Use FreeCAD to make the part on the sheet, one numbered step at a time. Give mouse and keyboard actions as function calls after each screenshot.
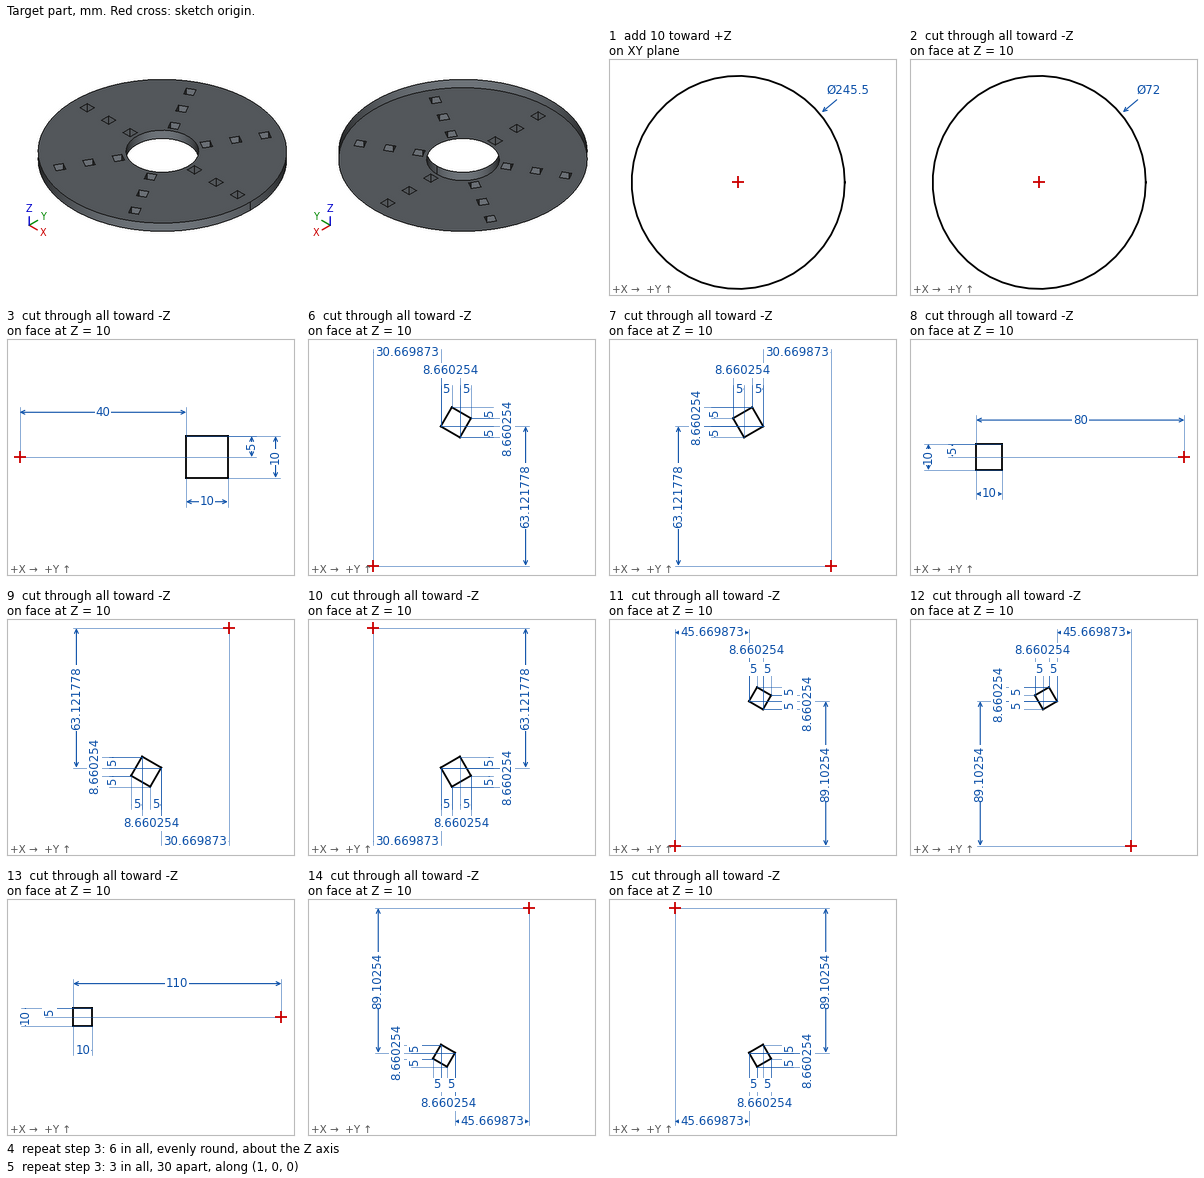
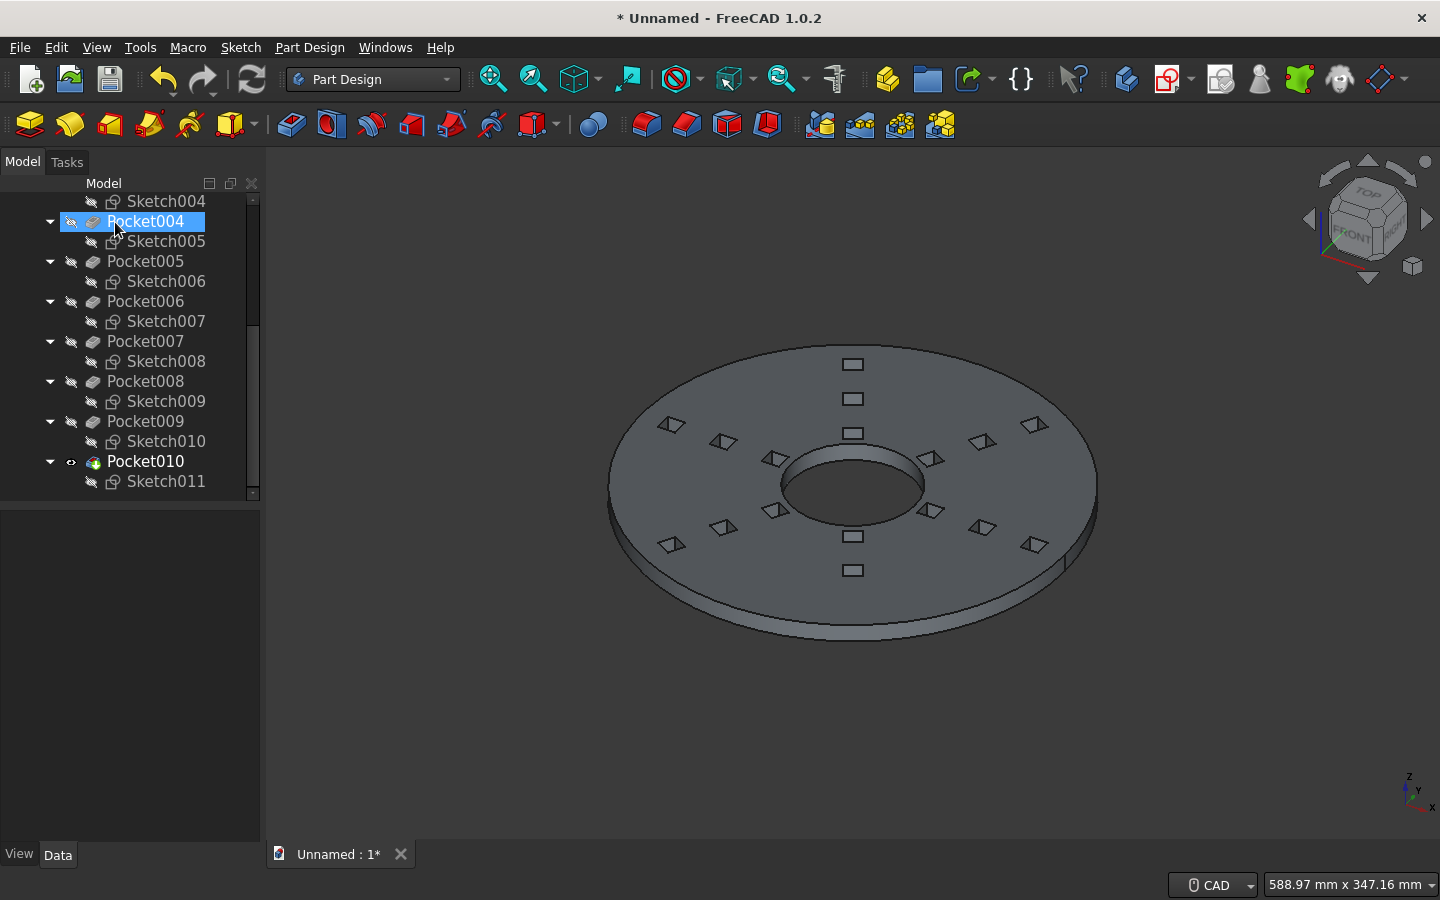
click(923, 414)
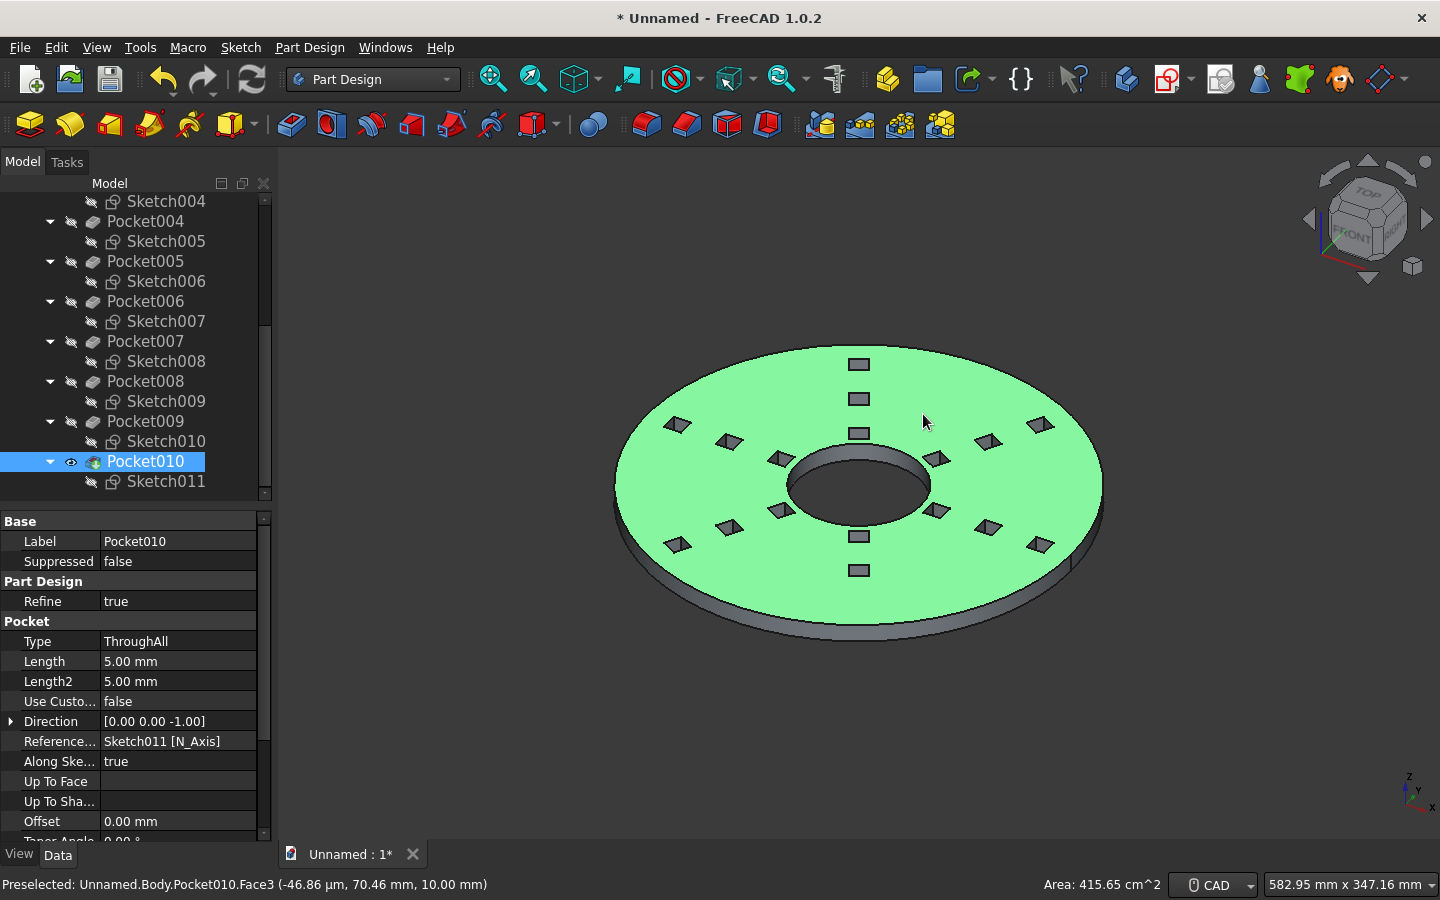
click(1168, 80)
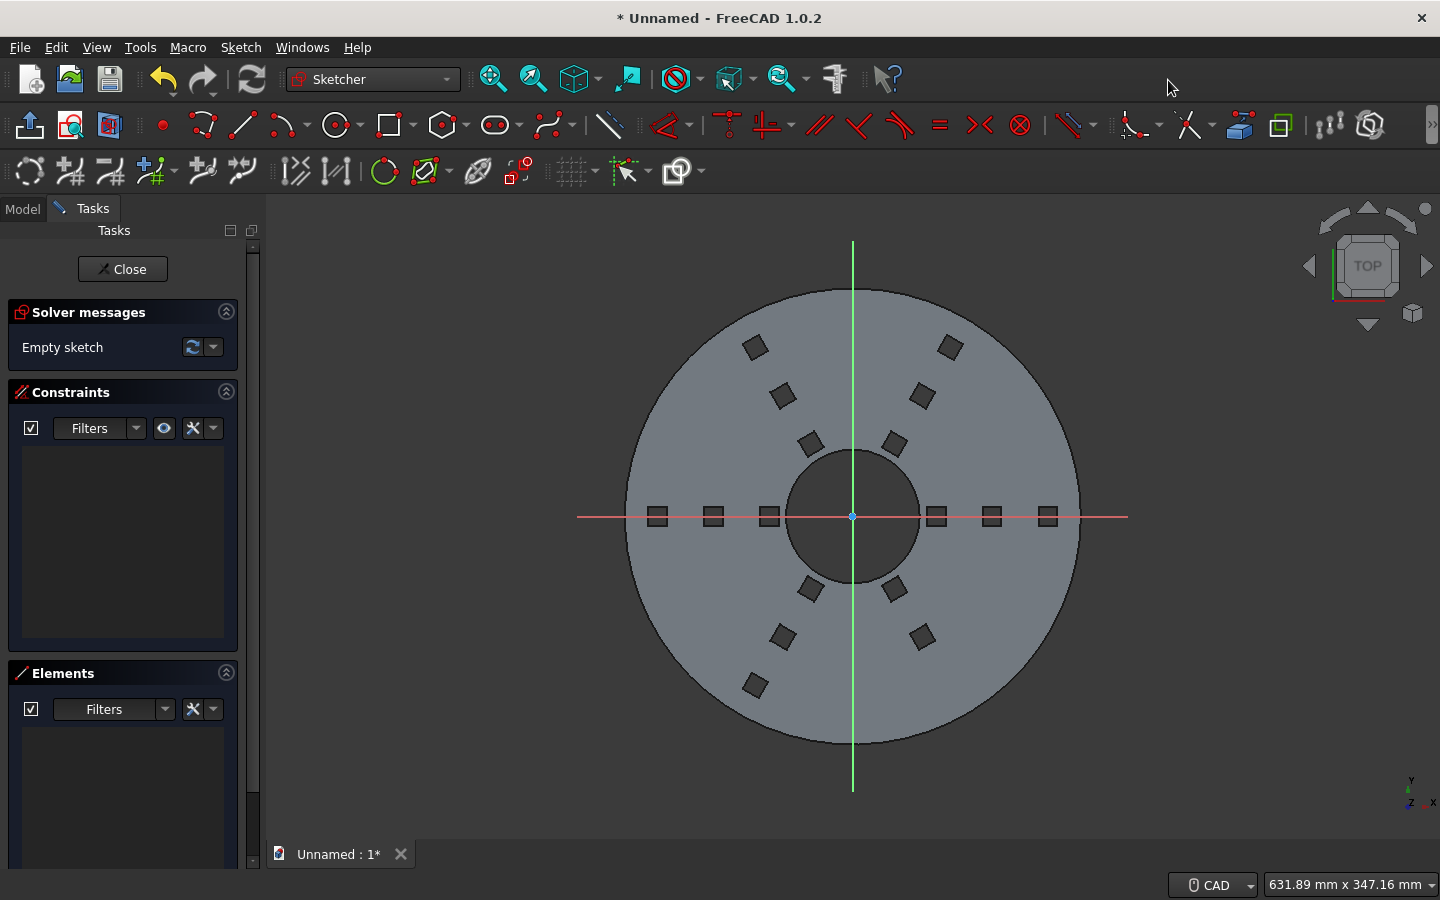
scroll(961, 696, up, 14)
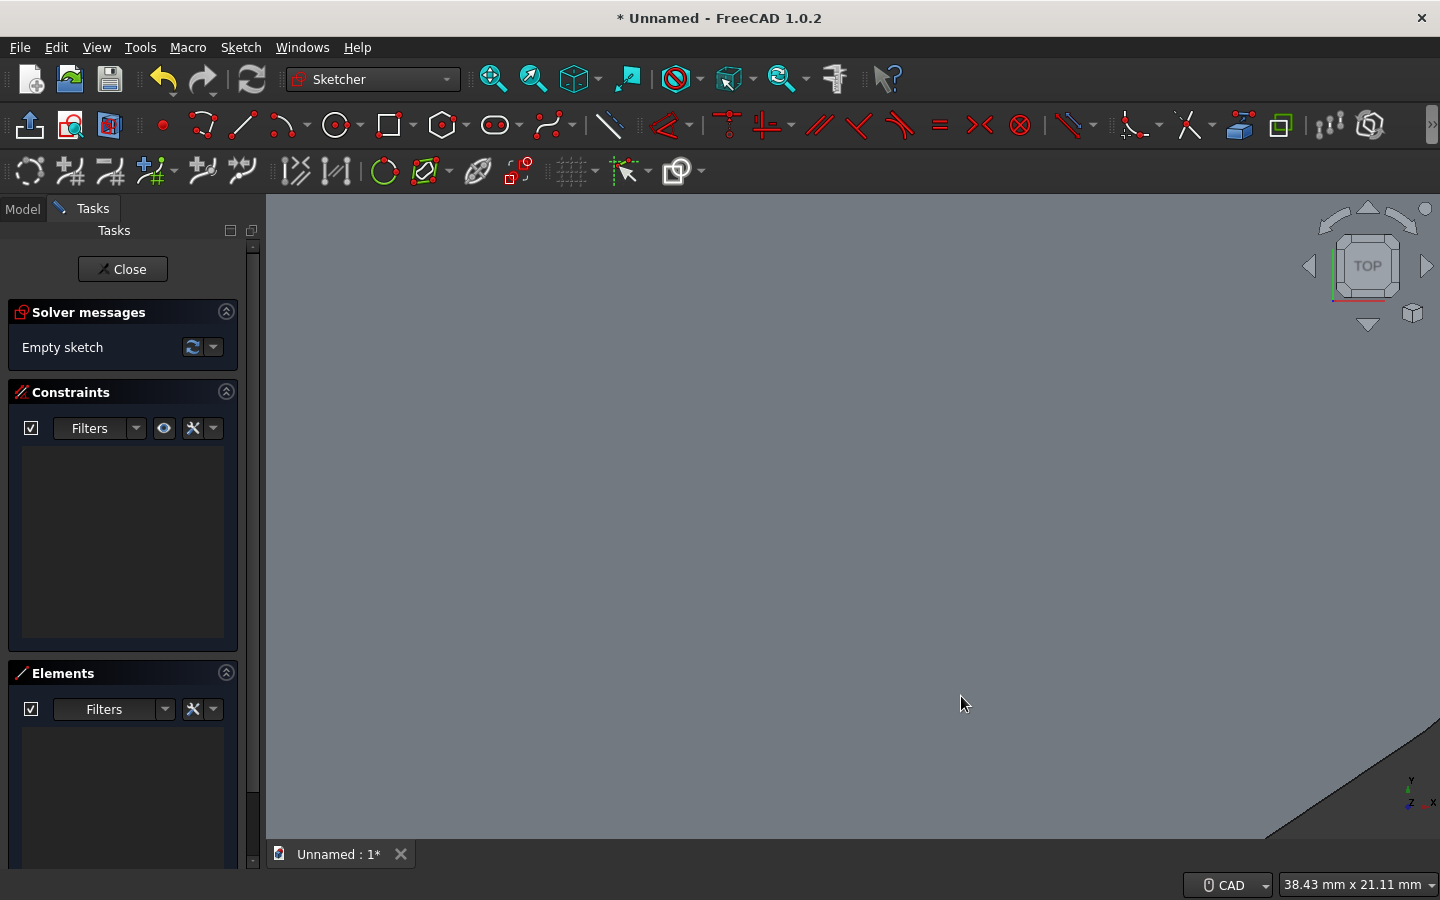
click(204, 126)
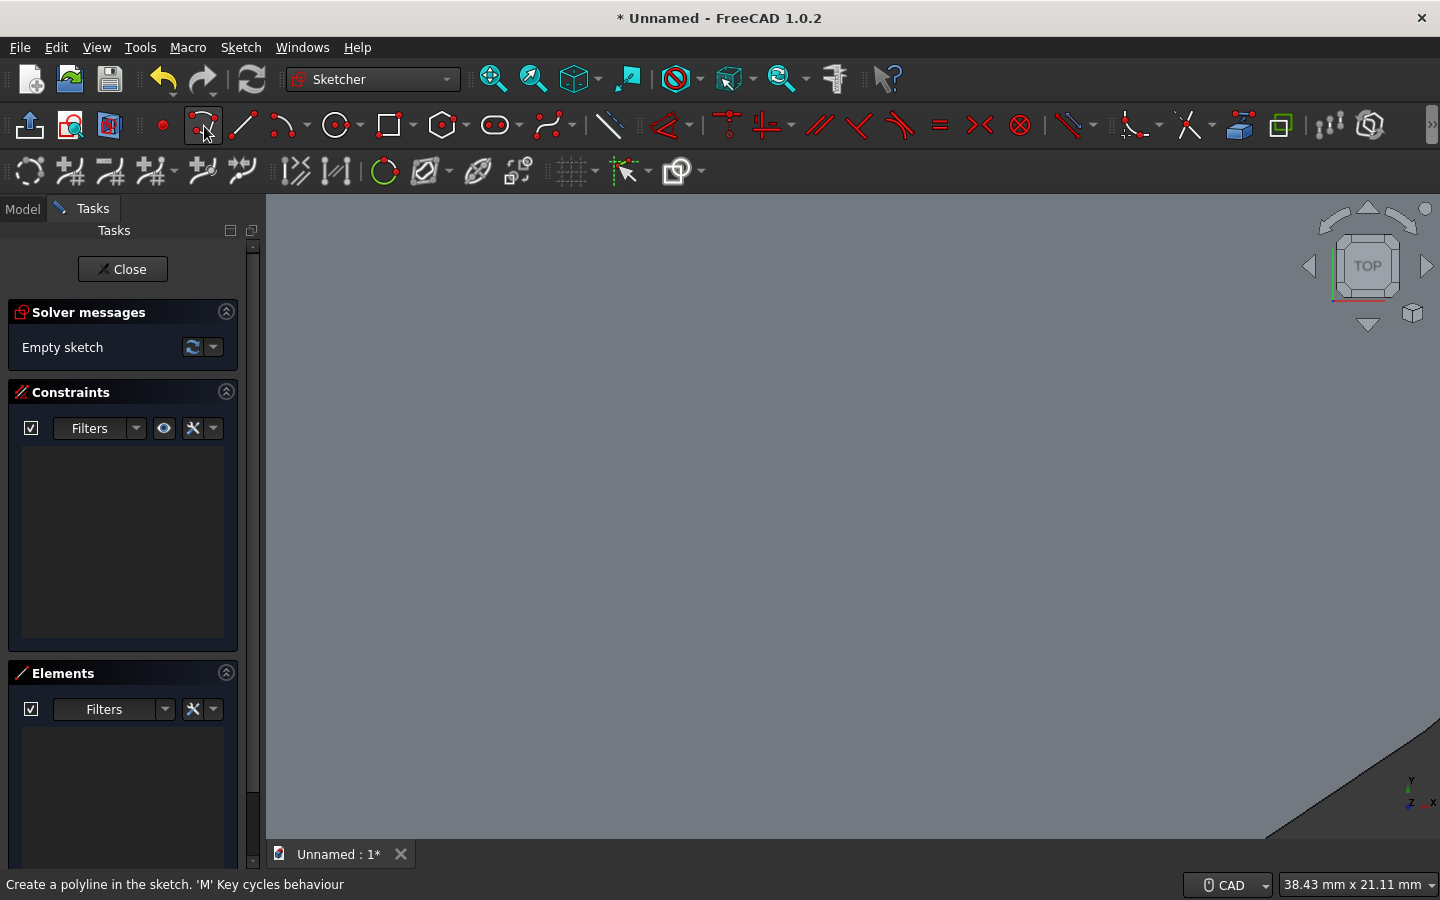
click(569, 454)
click(721, 719)
click(986, 566)
click(833, 302)
click(569, 455)
key(Escape)
key(Escape)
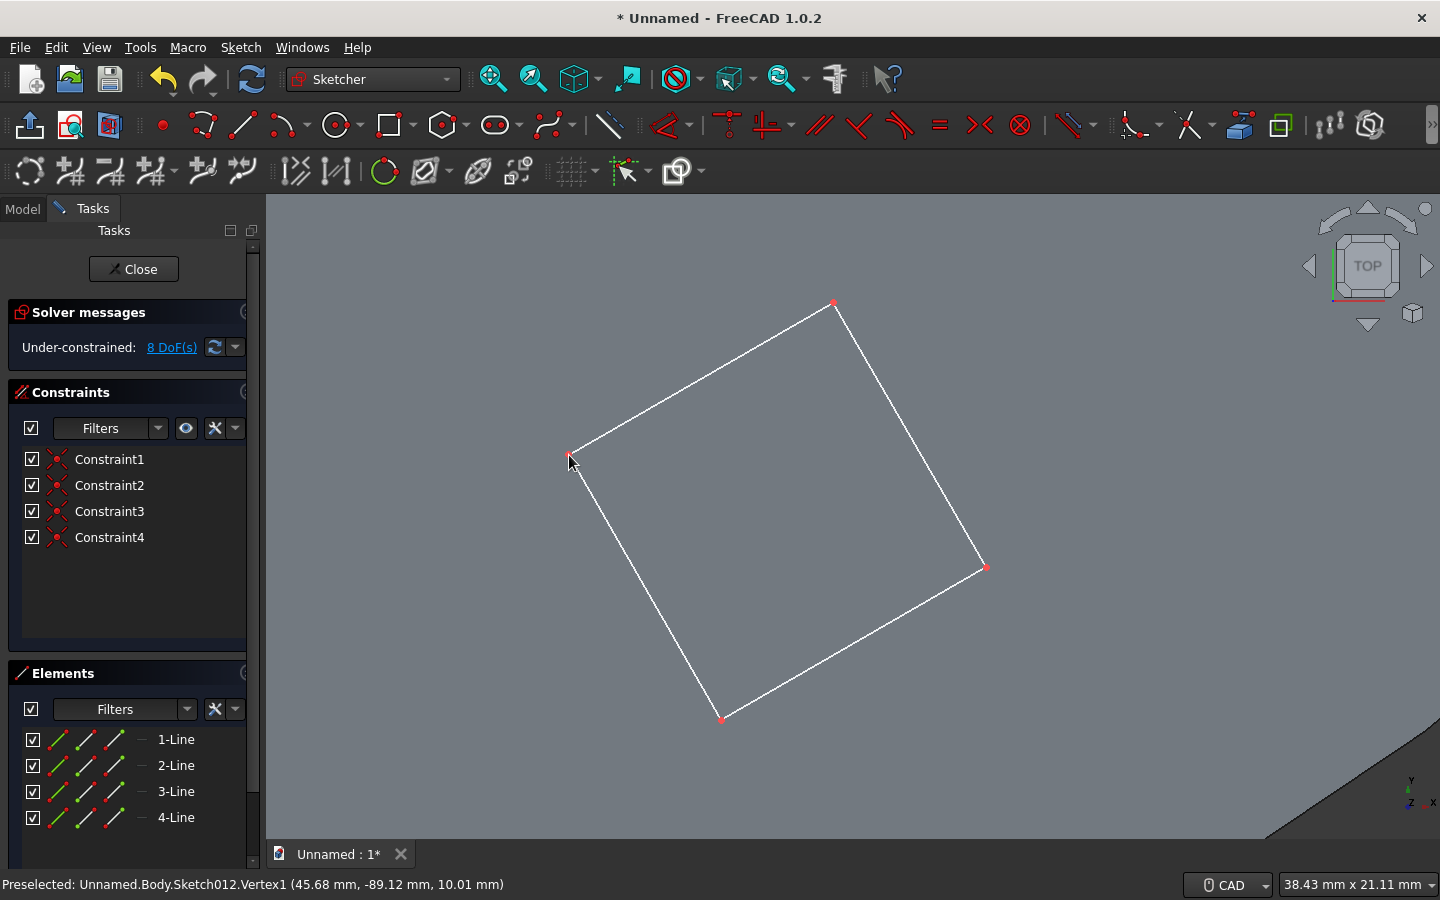
key(d)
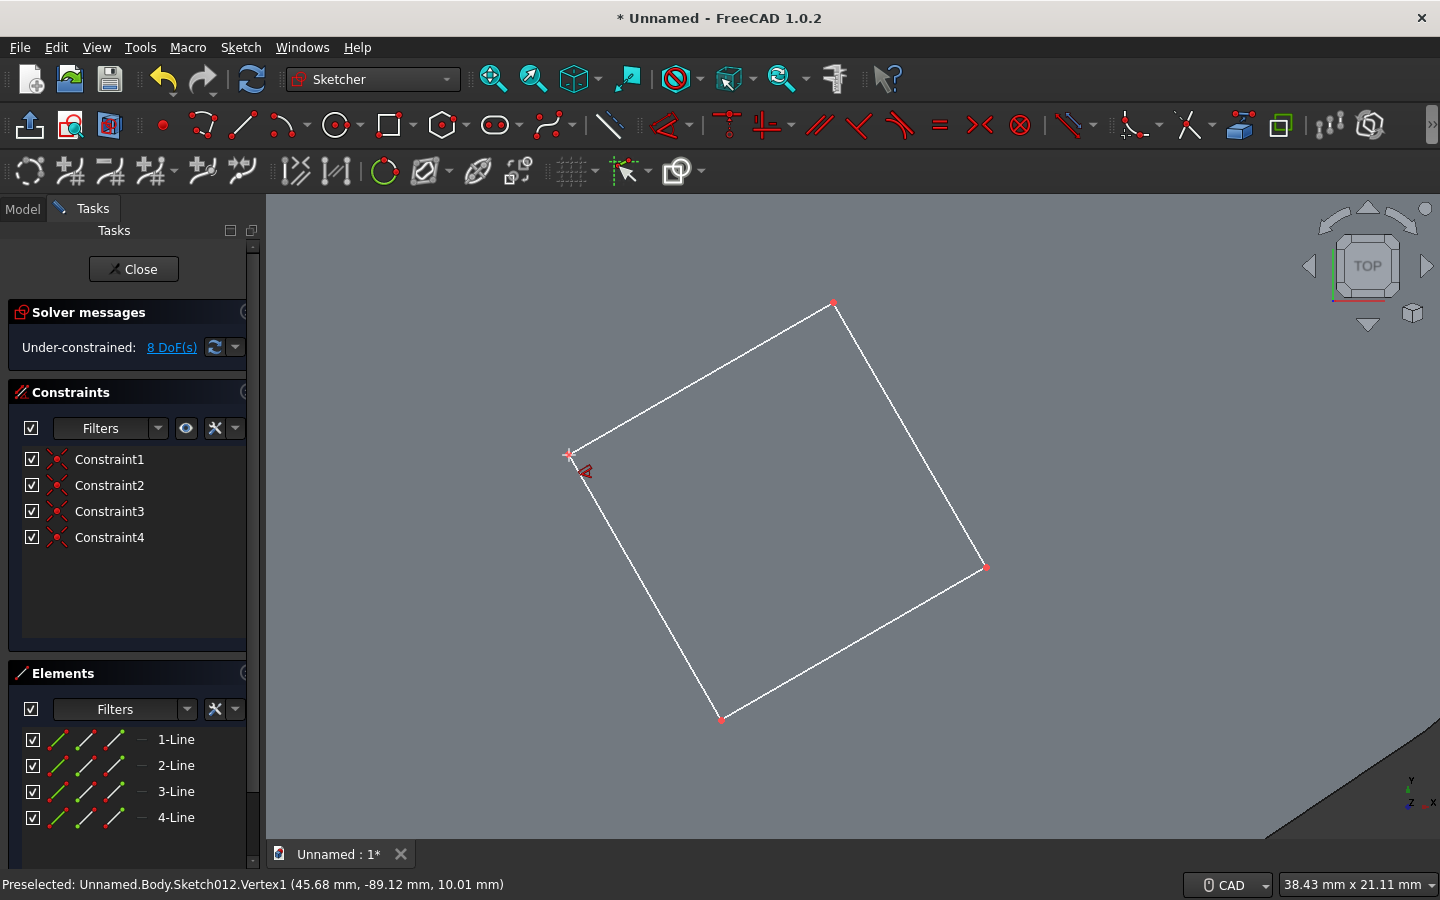
click(615, 534)
click(645, 754)